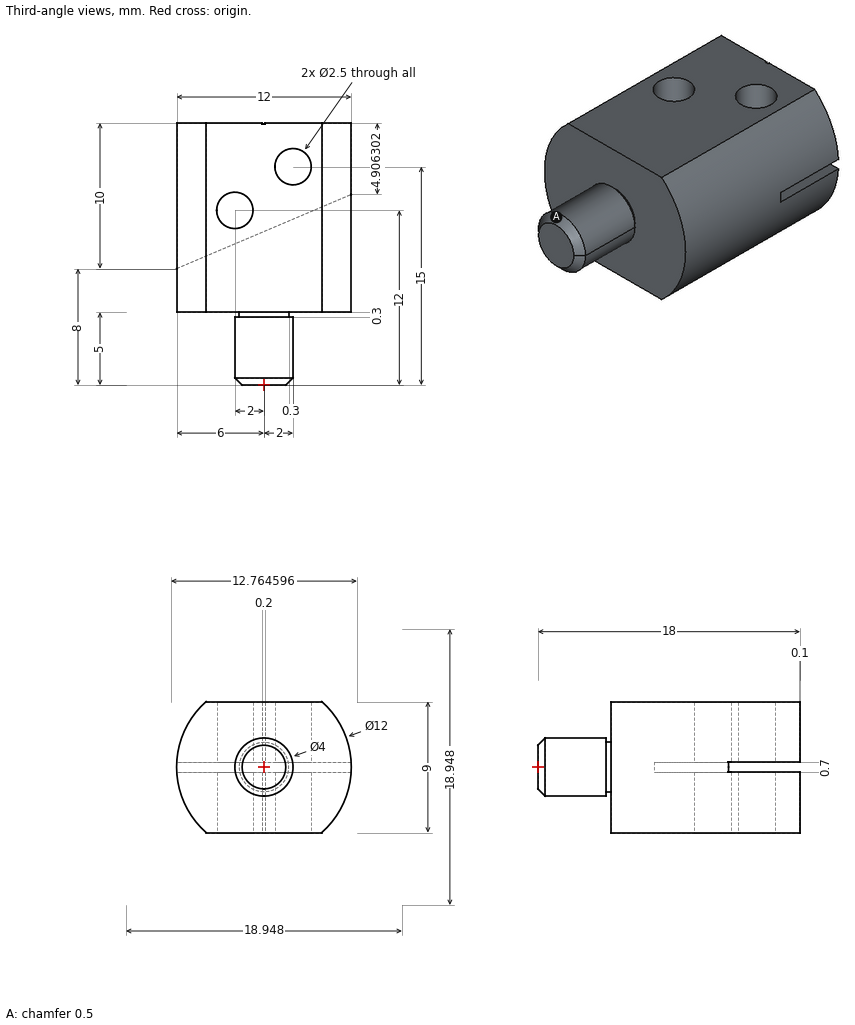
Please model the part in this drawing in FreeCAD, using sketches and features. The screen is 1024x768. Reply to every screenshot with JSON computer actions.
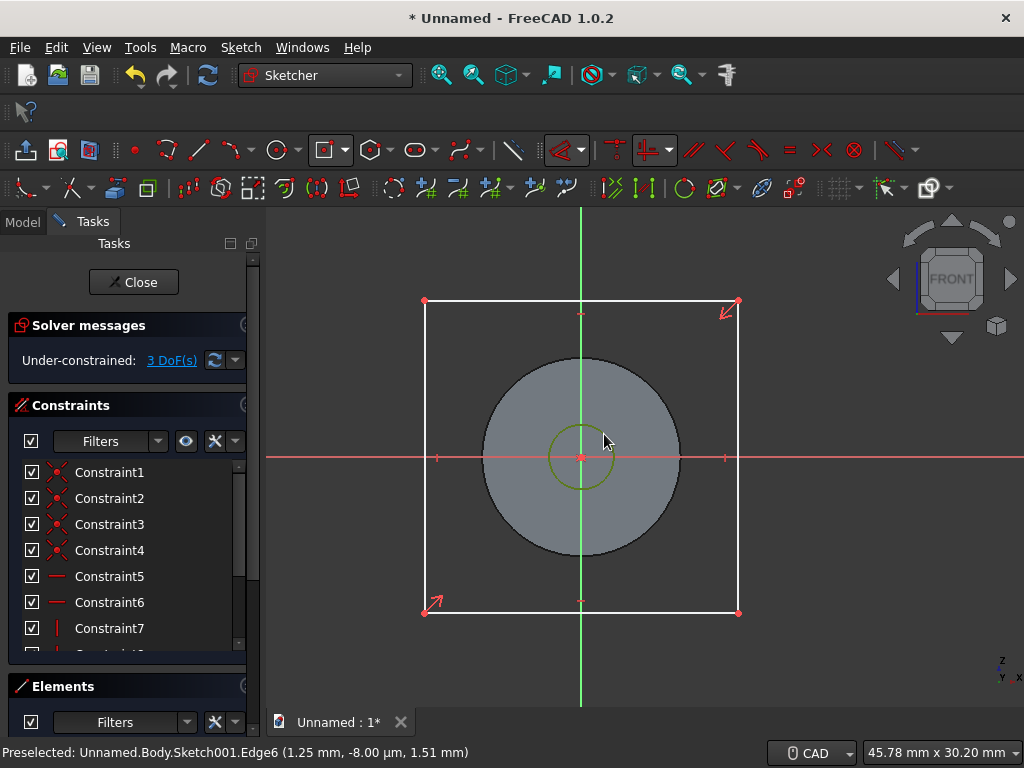
{"action": "left_click", "coordinate": [584, 150]}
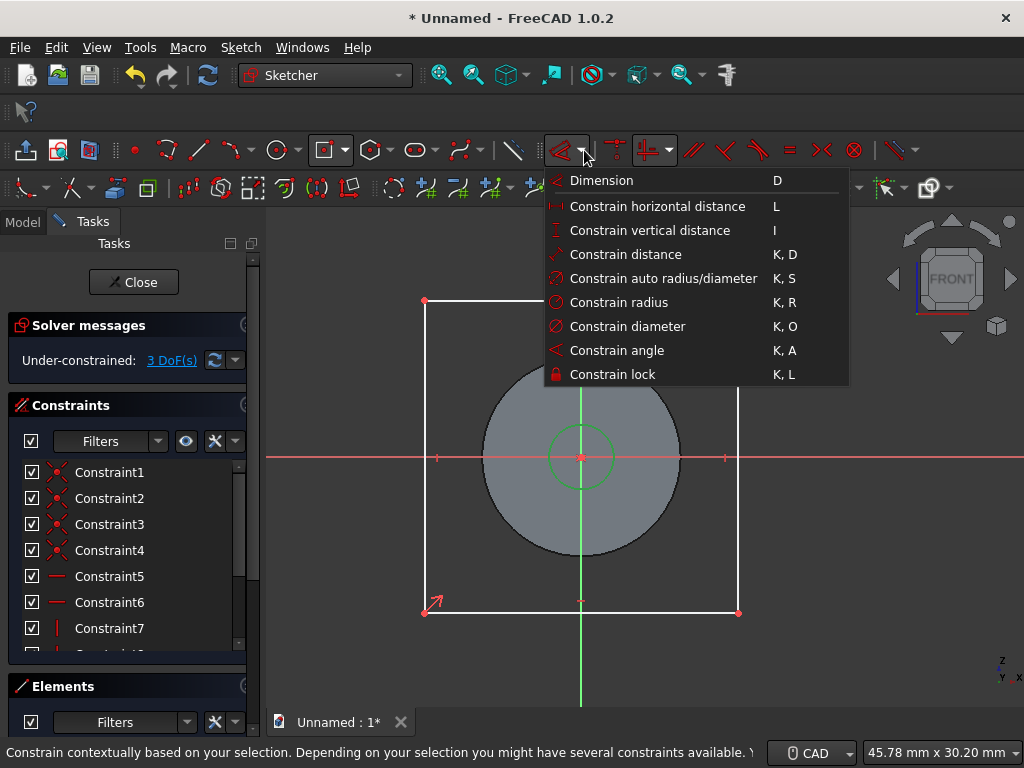
{"action": "left_click", "coordinate": [697, 326]}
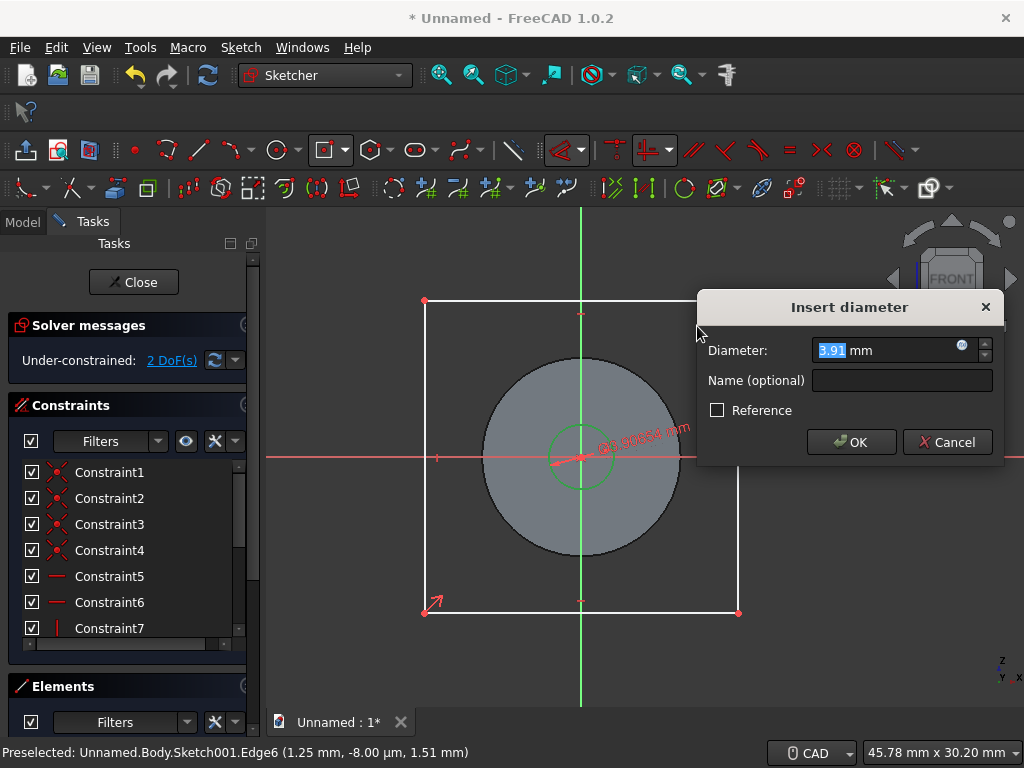
{"action": "type", "text": "4"}
{"action": "key", "text": "Return"}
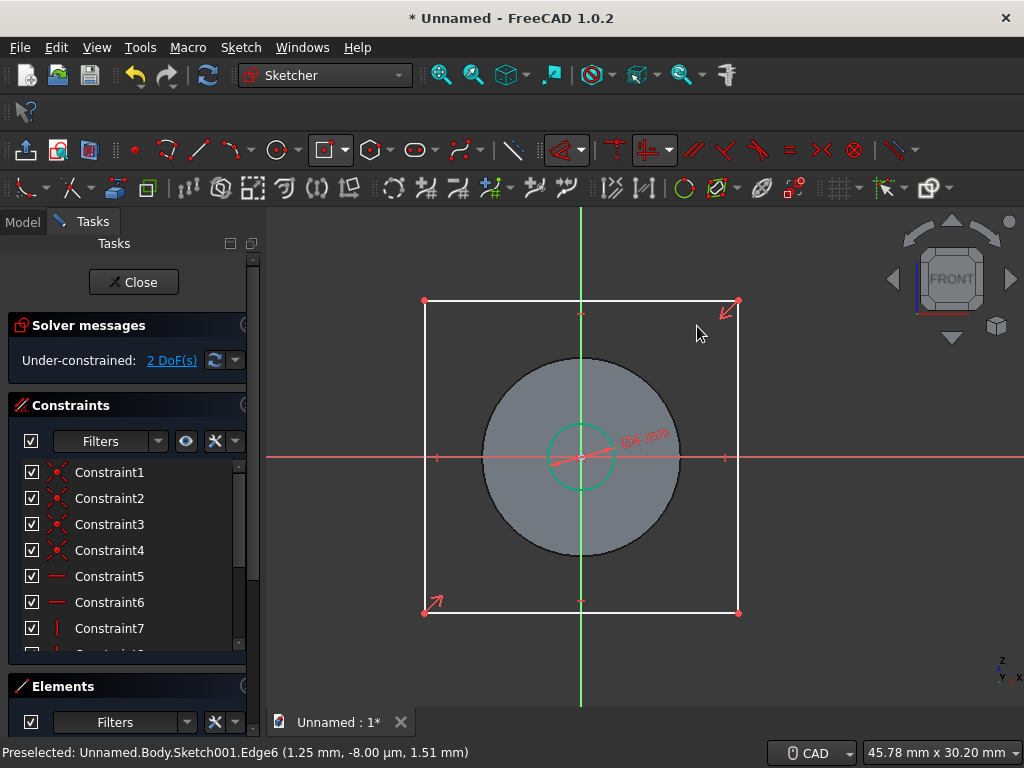
{"action": "left_click", "coordinate": [519, 613]}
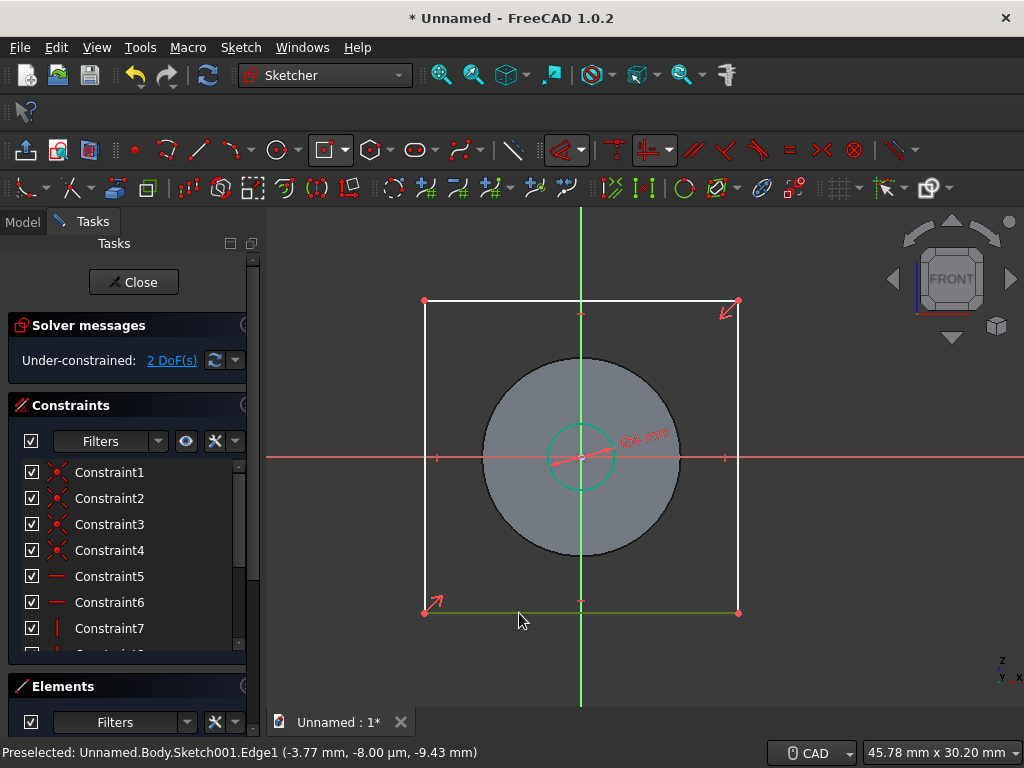
{"action": "key", "text": "l"}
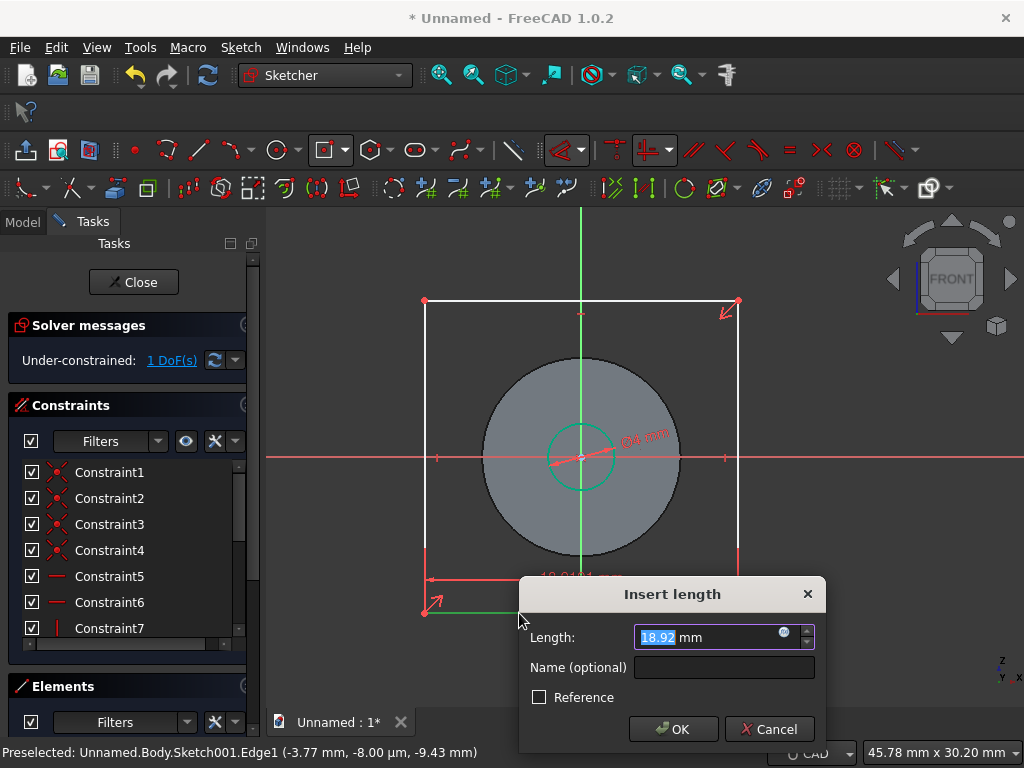
{"action": "type", "text": "18.948"}
{"action": "key", "text": "Return"}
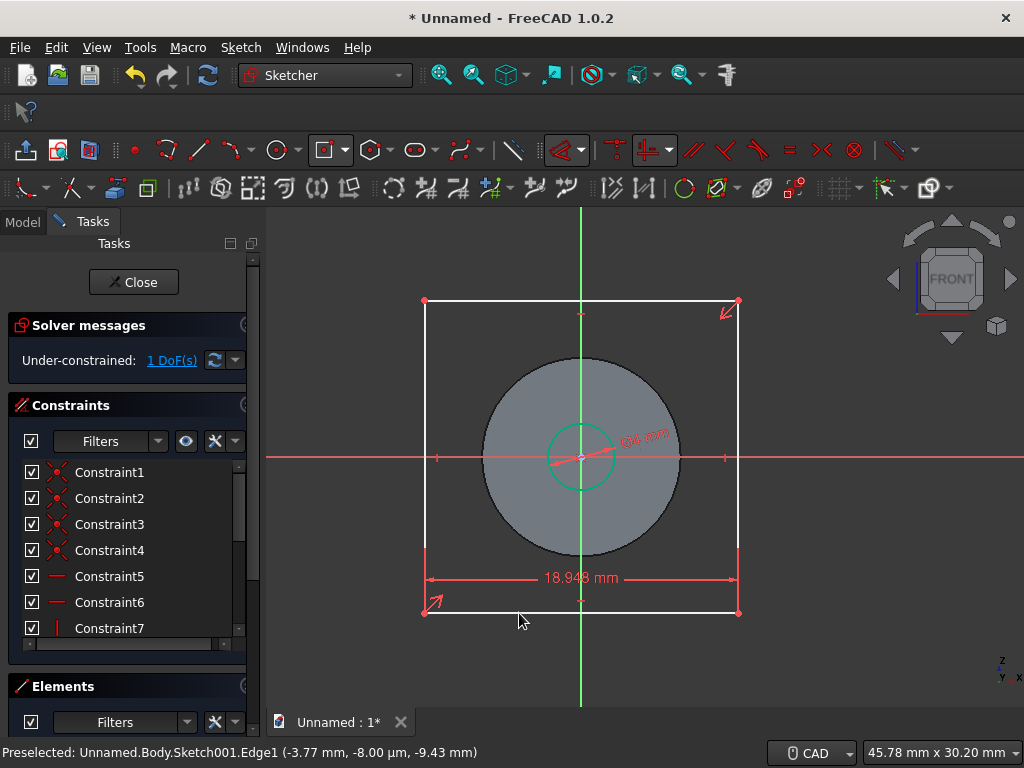
{"action": "left_click", "coordinate": [738, 520]}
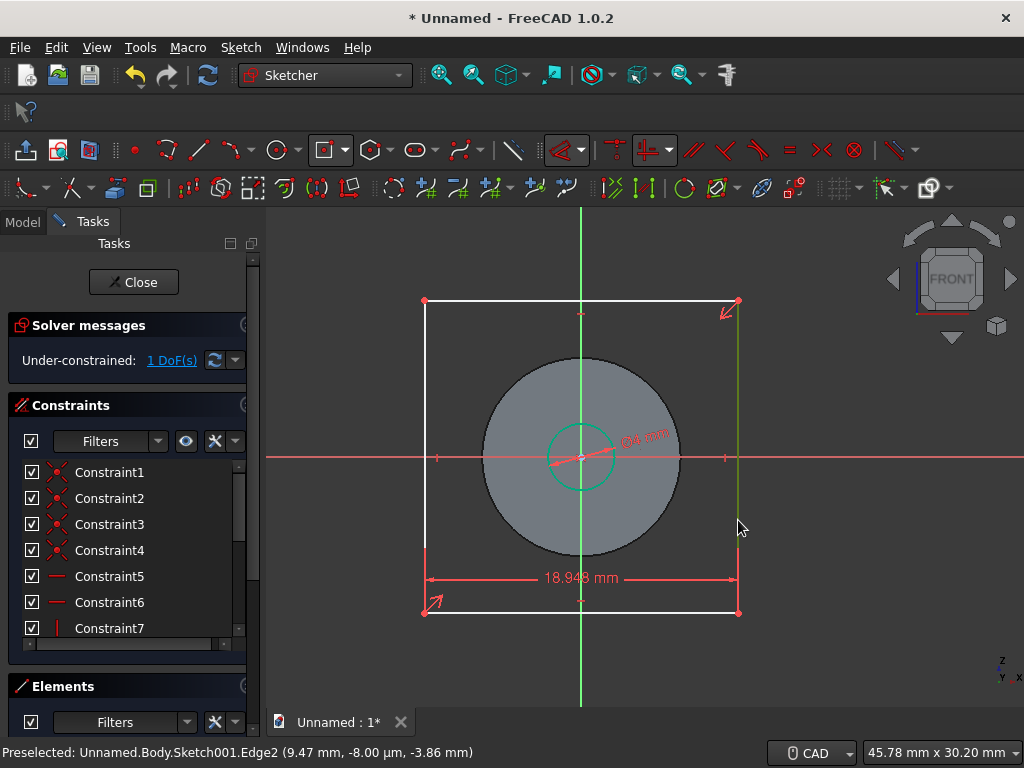
{"action": "left_click", "coordinate": [584, 150]}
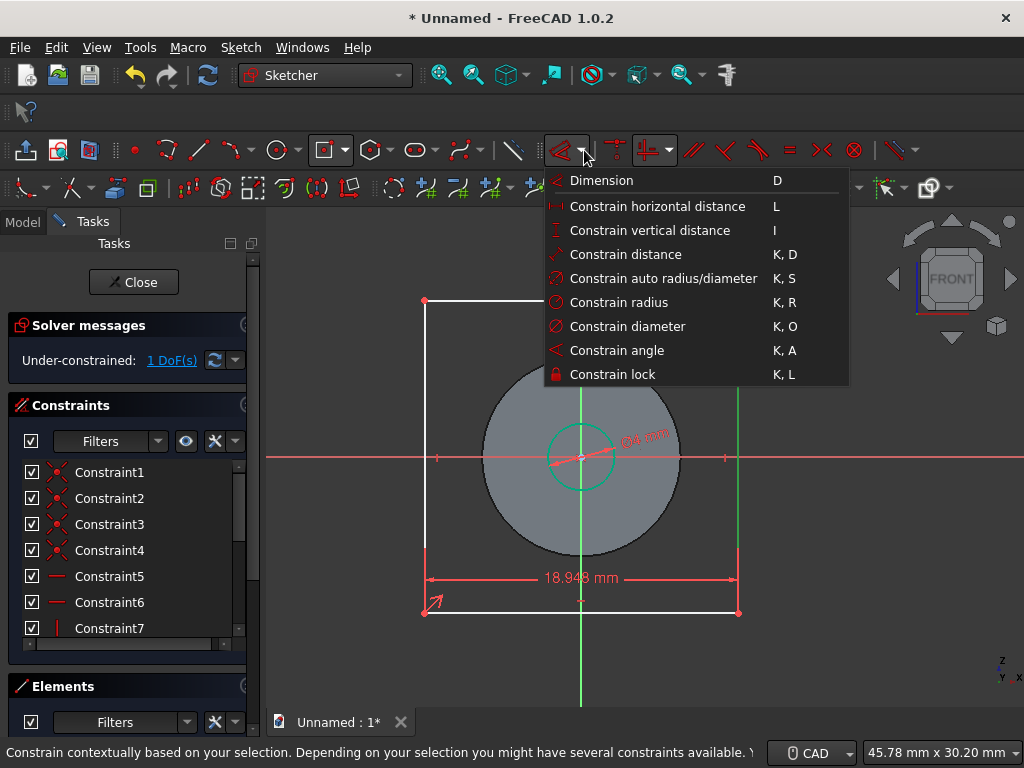
{"action": "left_click", "coordinate": [697, 230]}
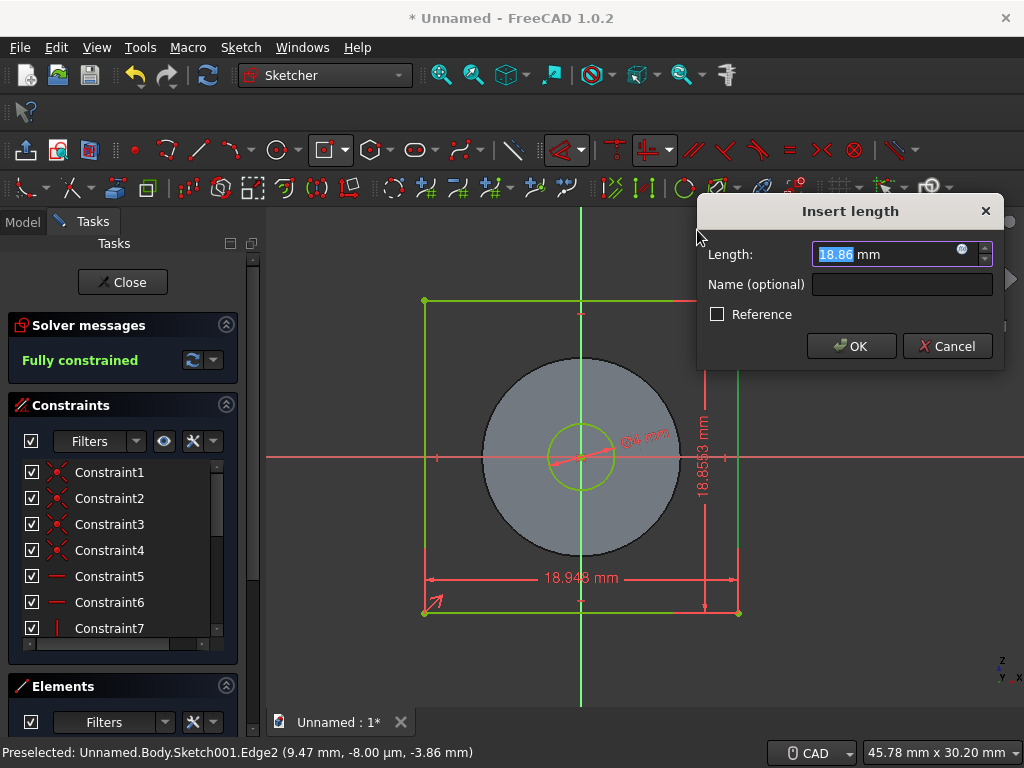
{"action": "type", "text": "18.948"}
{"action": "key", "text": "Return"}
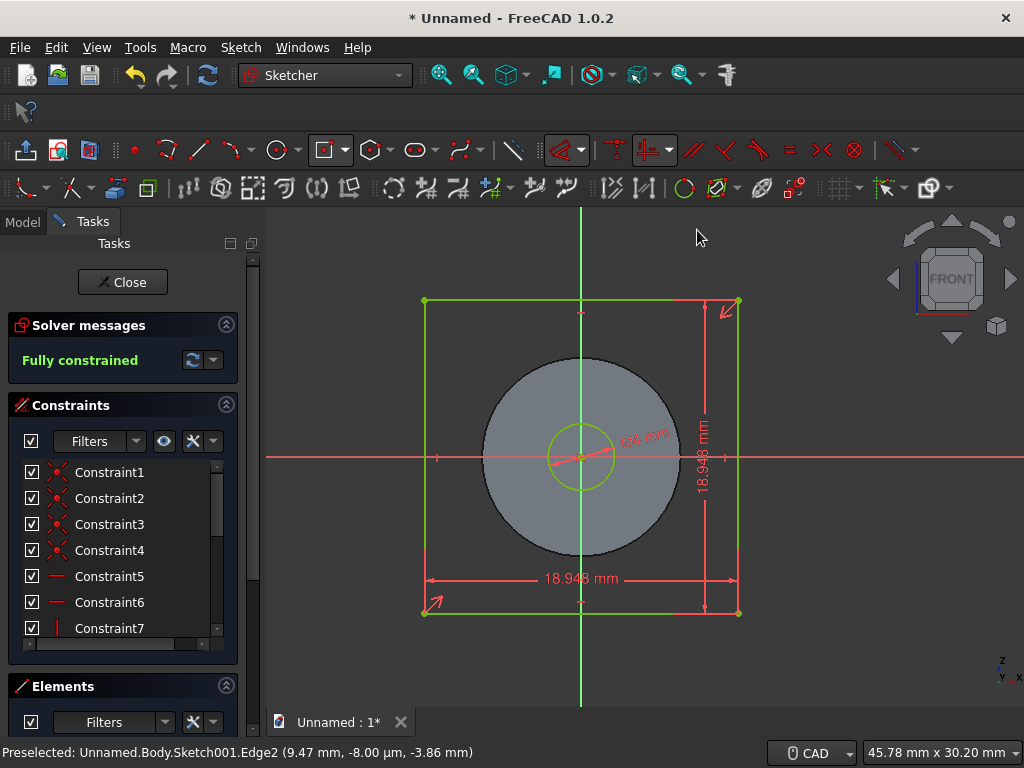
{"action": "left_click", "coordinate": [123, 282]}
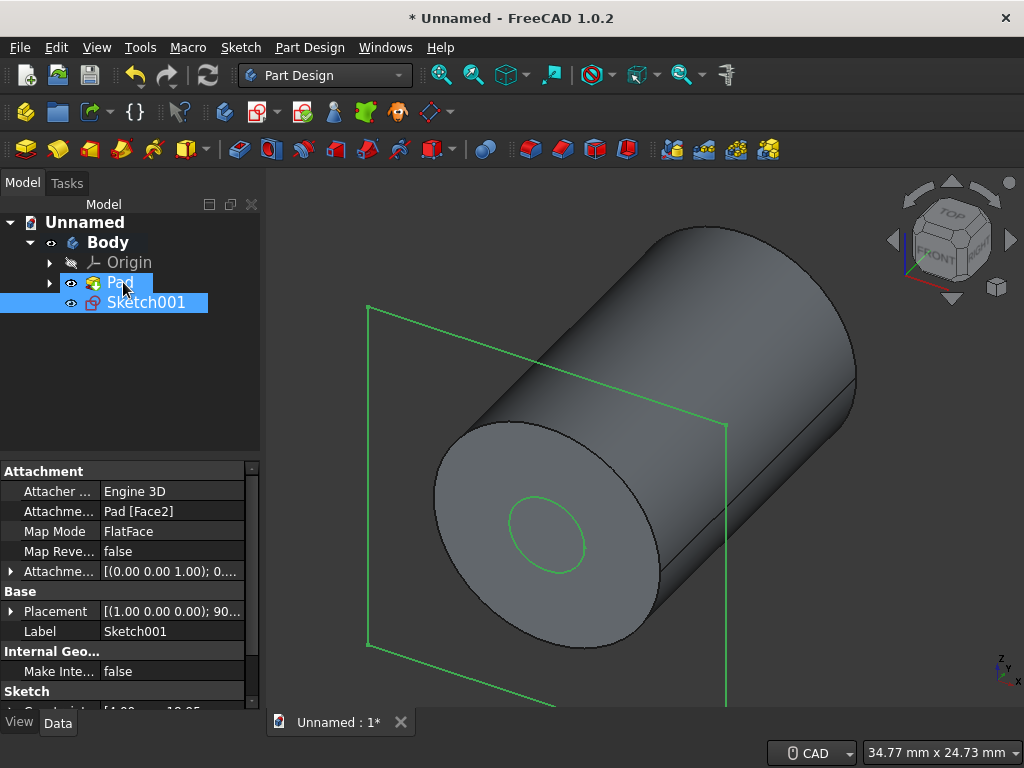
{"action": "left_click", "coordinate": [240, 150]}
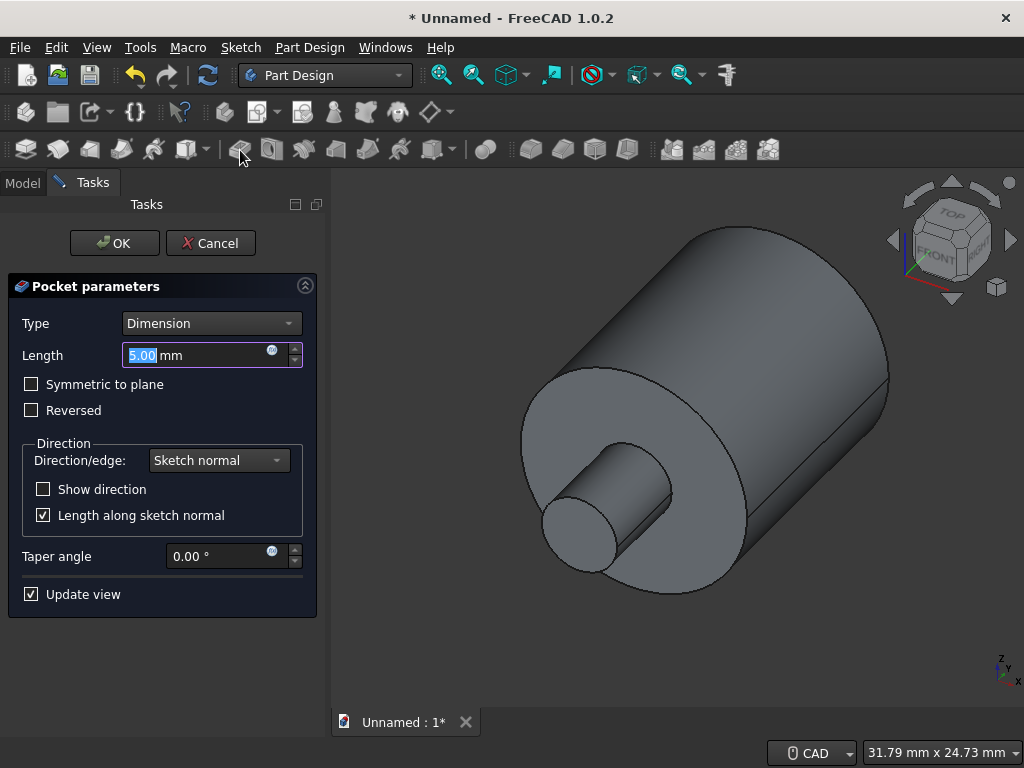
{"action": "type", "text": "5"}
{"action": "key", "text": "Tab"}